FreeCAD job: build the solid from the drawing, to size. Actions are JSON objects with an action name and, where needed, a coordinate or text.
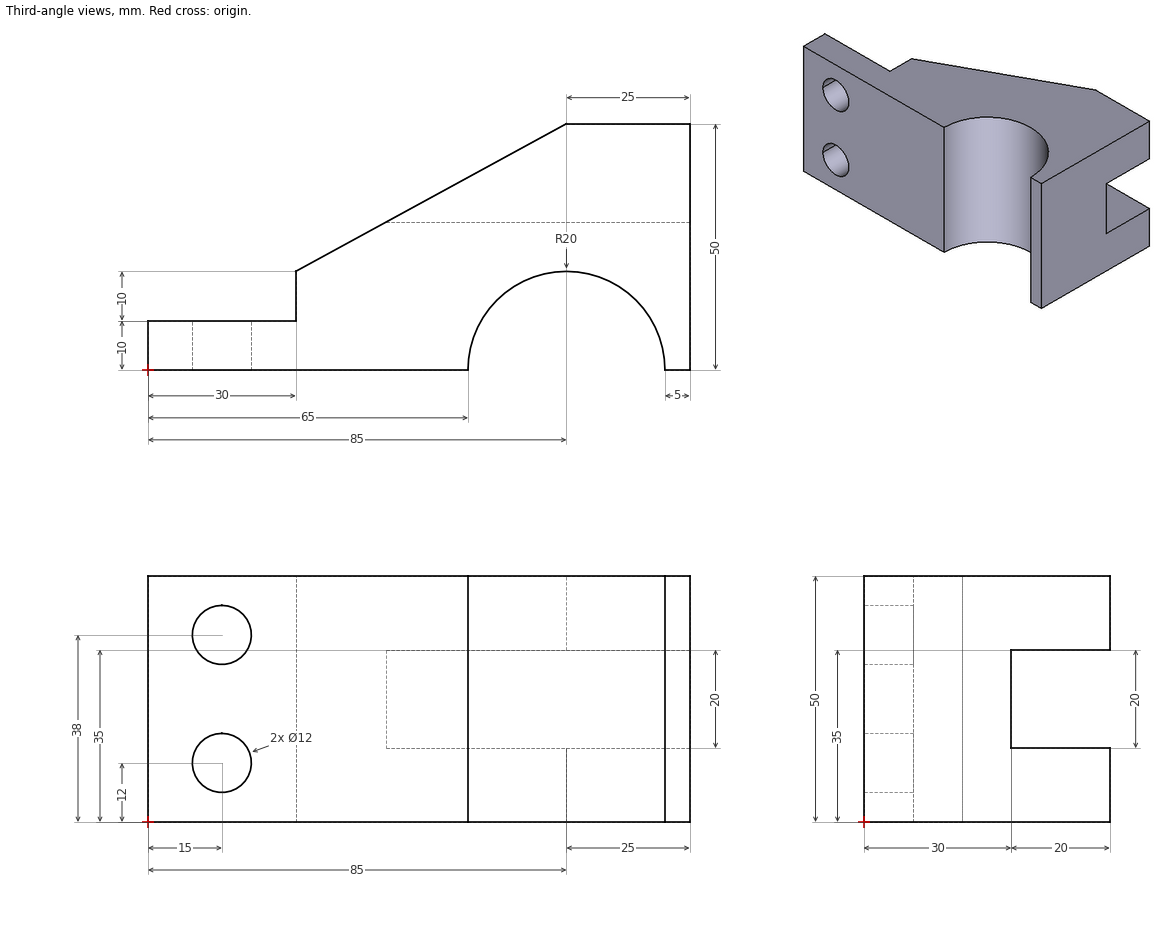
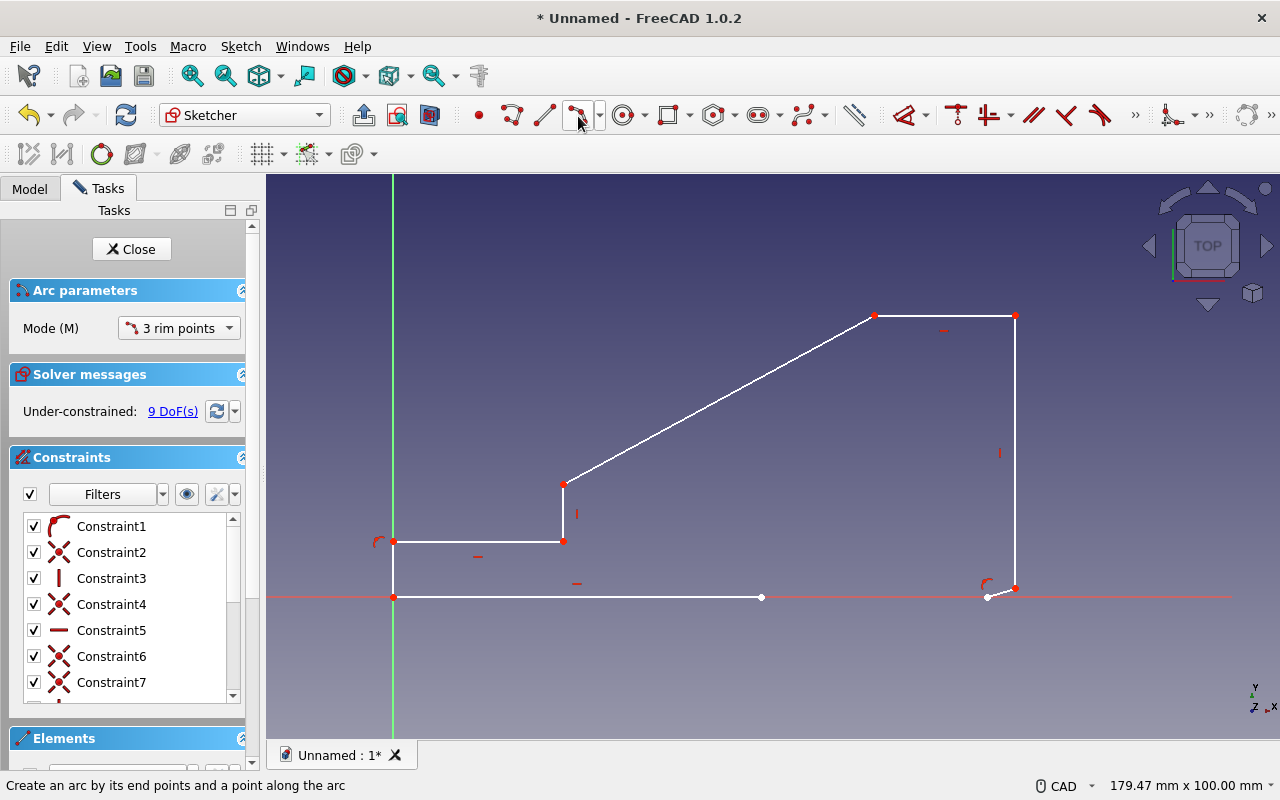
{"action": "left_click", "coordinate": [761, 588]}
{"action": "left_click", "coordinate": [987, 597]}
{"action": "left_click", "coordinate": [874, 484]}
{"action": "key", "text": "Escape"}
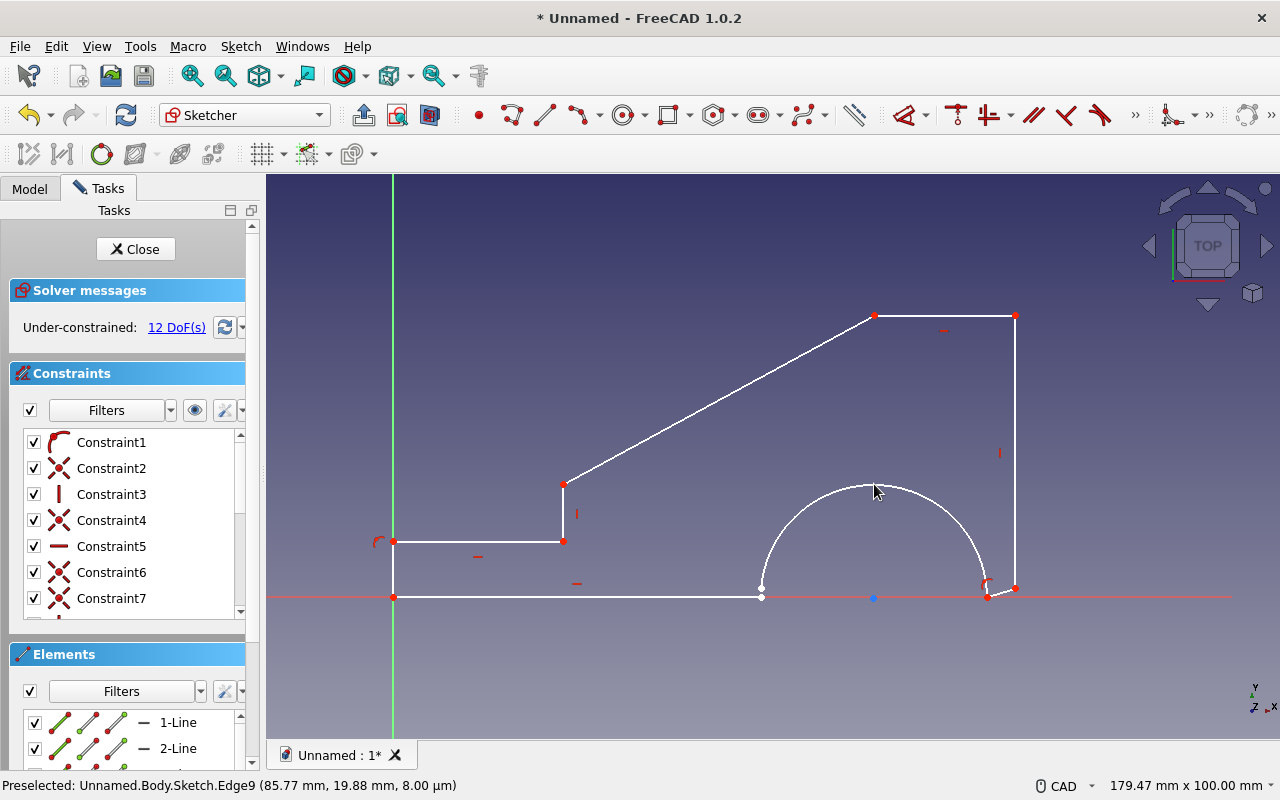
{"action": "scroll", "coordinate": [998, 594], "scroll_direction": "up", "scroll_amount": 2}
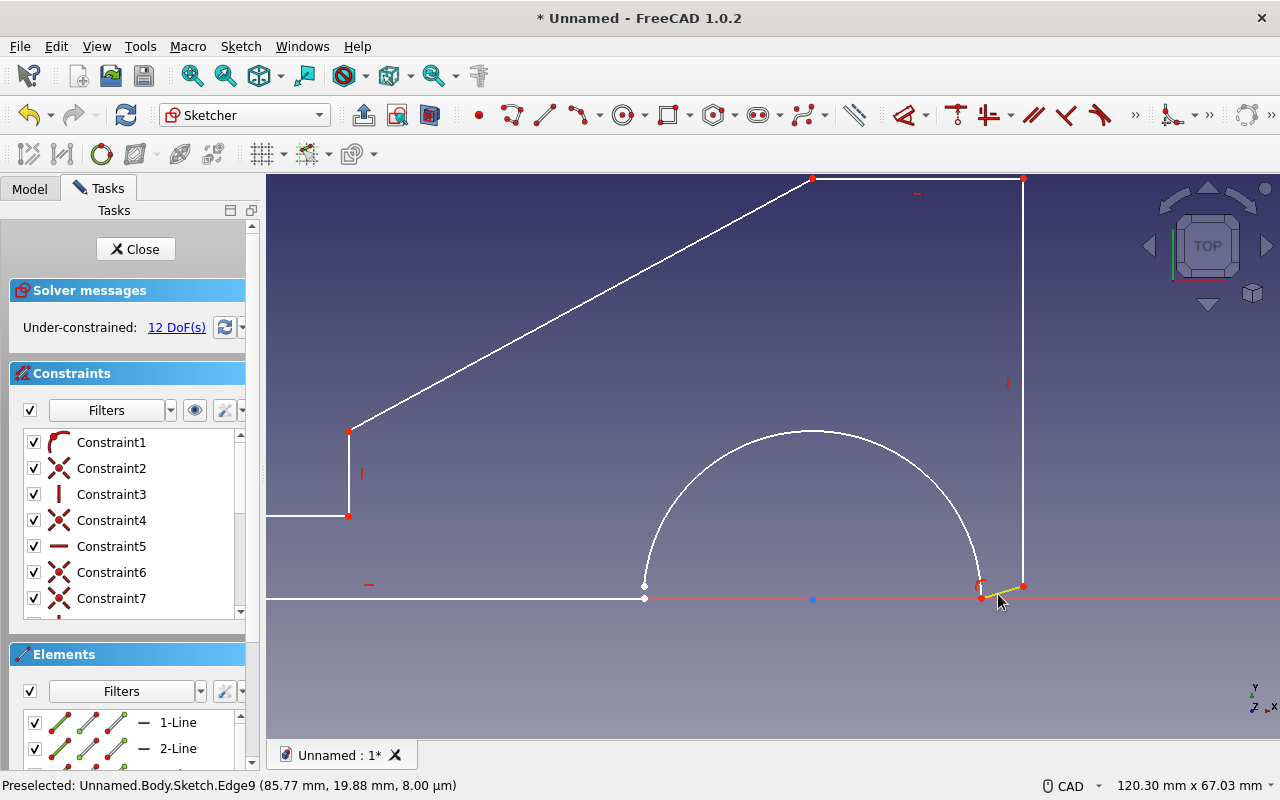
{"action": "left_click", "coordinate": [998, 594]}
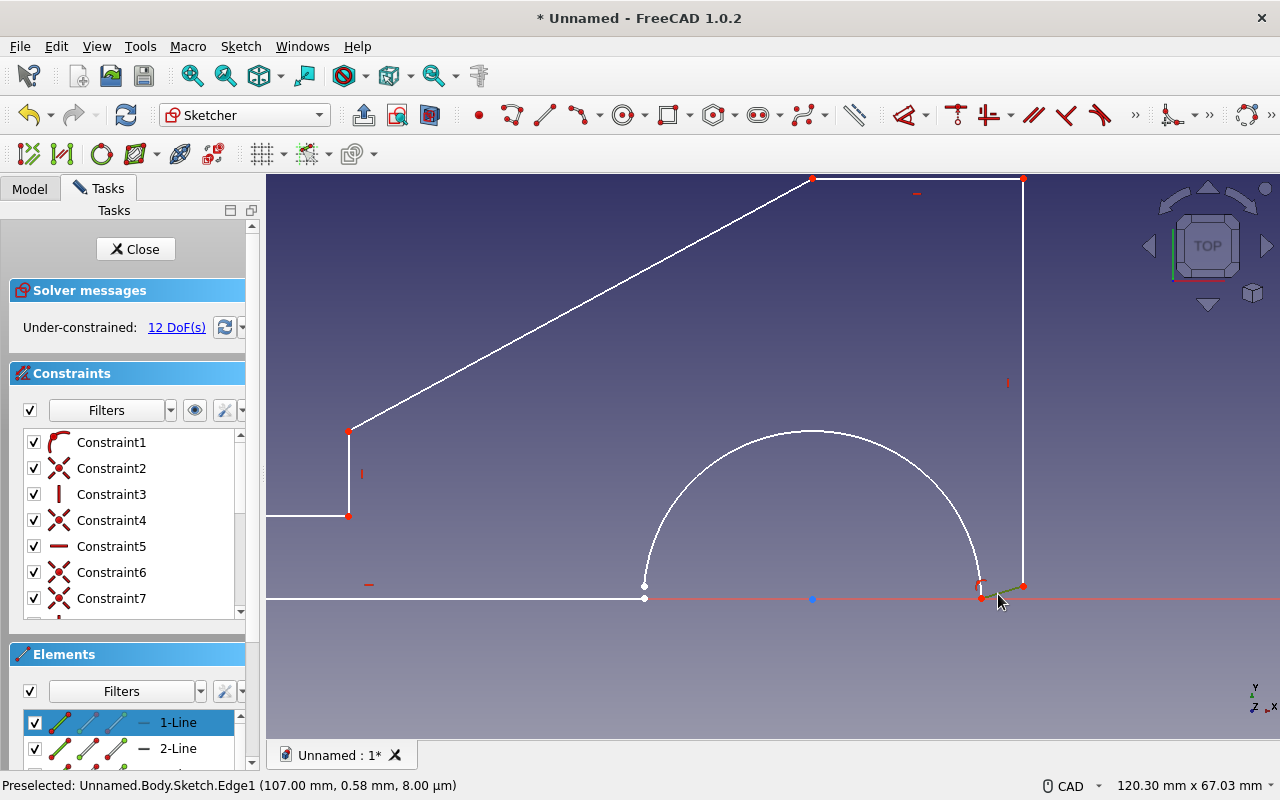
{"action": "left_click", "coordinate": [1010, 116]}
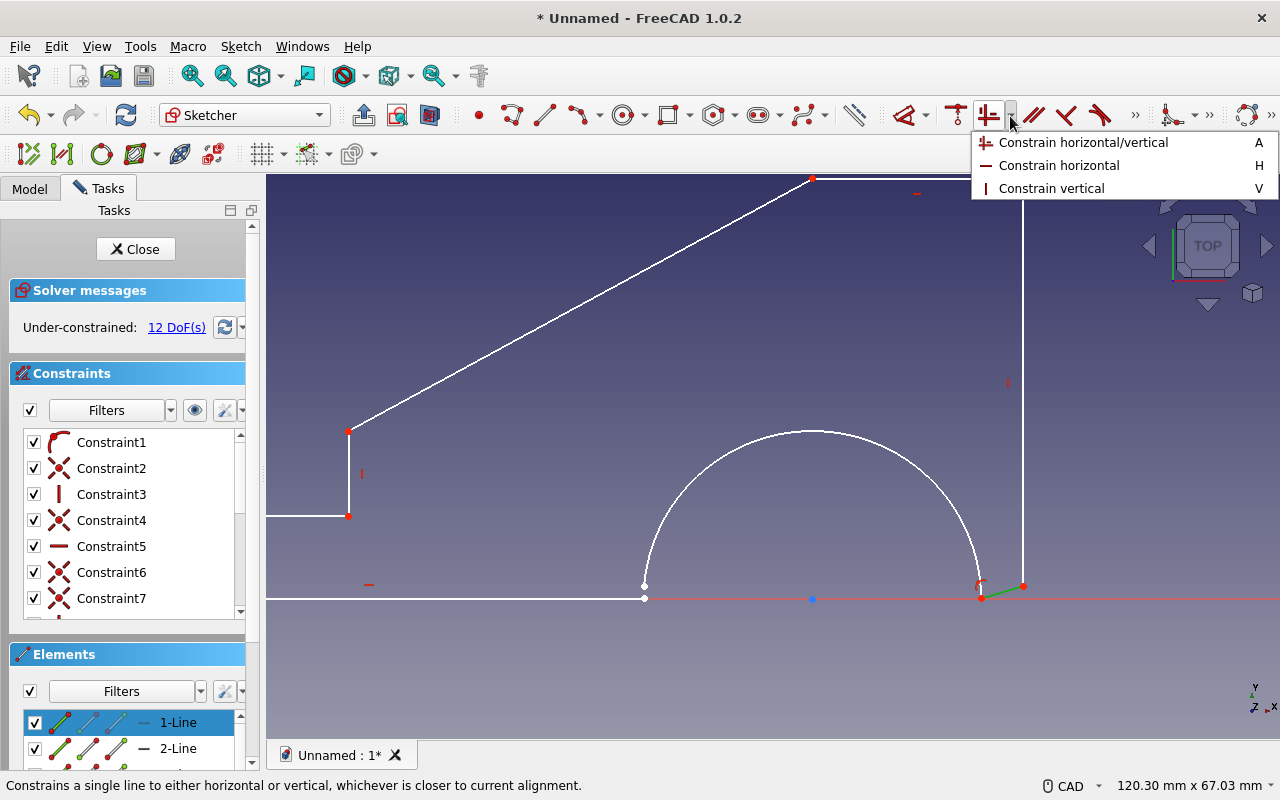
{"action": "left_click", "coordinate": [1125, 166]}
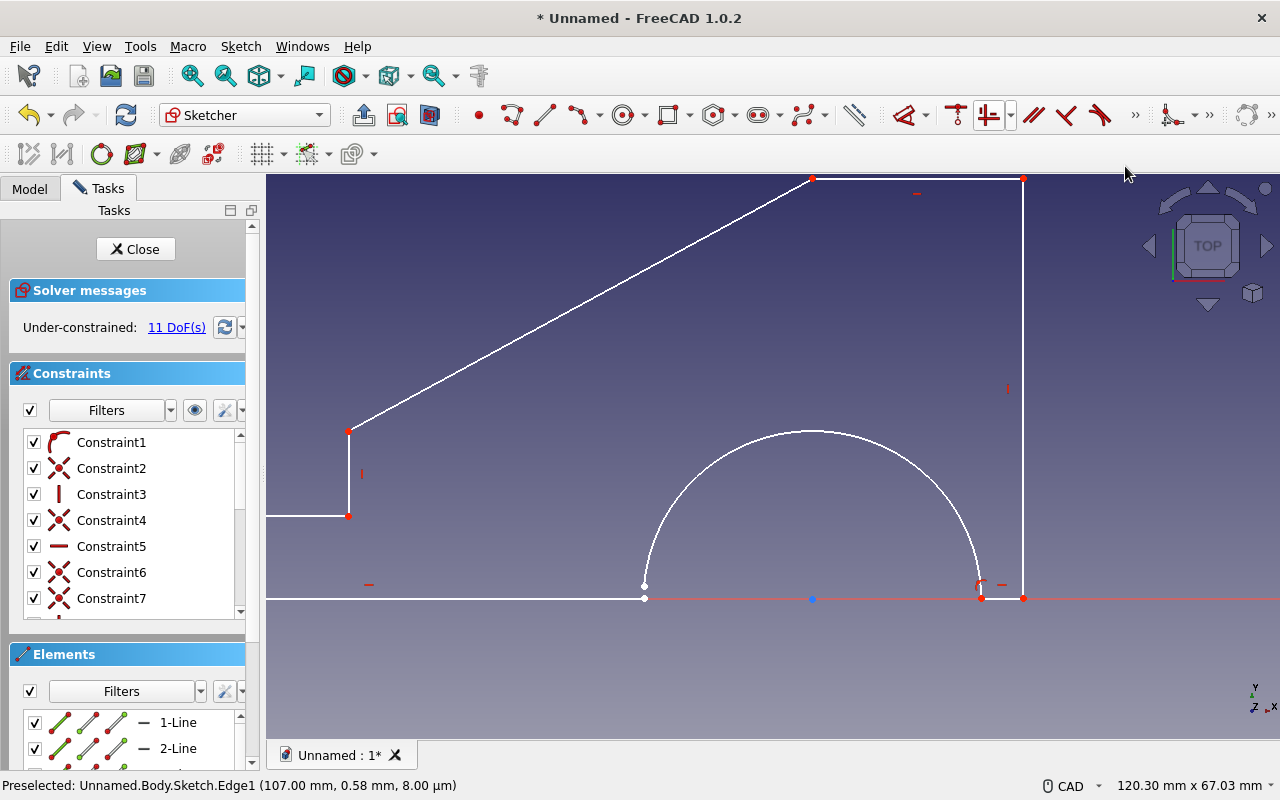
{"action": "left_click", "coordinate": [812, 600]}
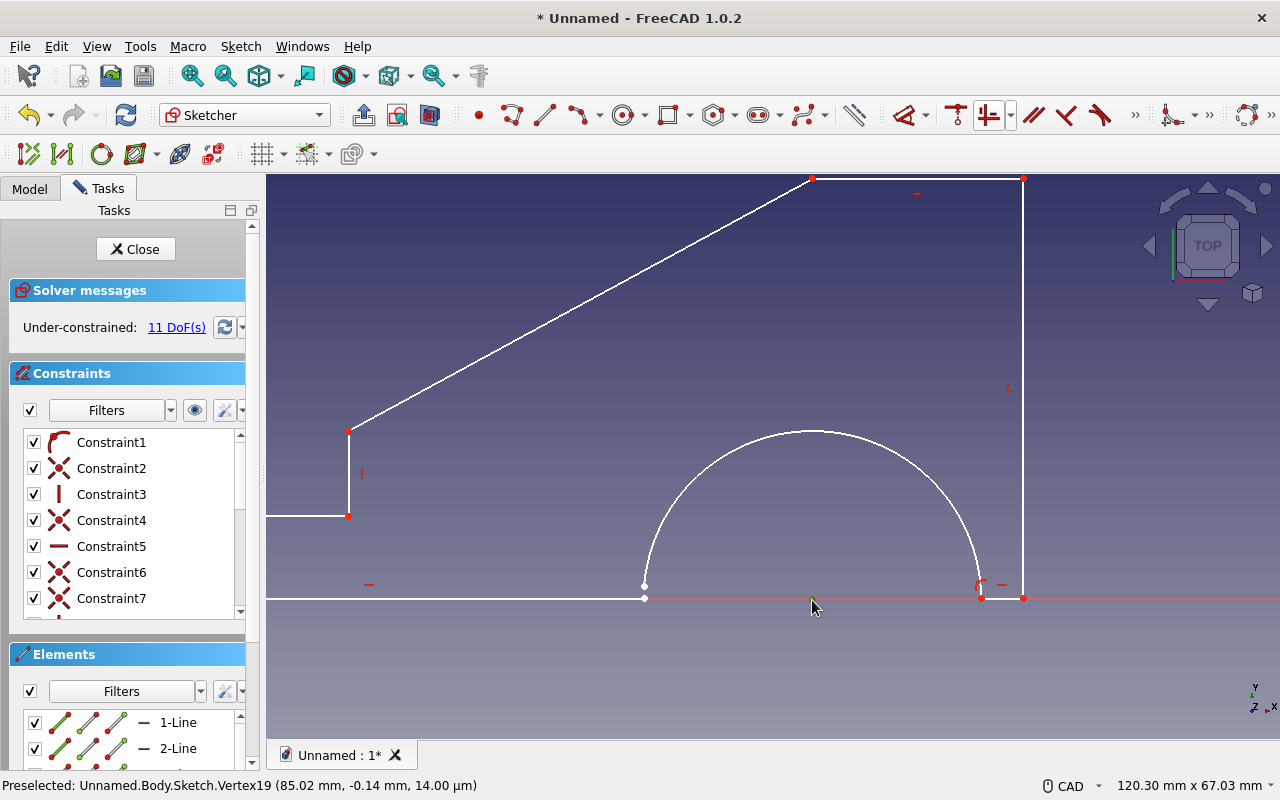
{"action": "left_click", "coordinate": [704, 599]}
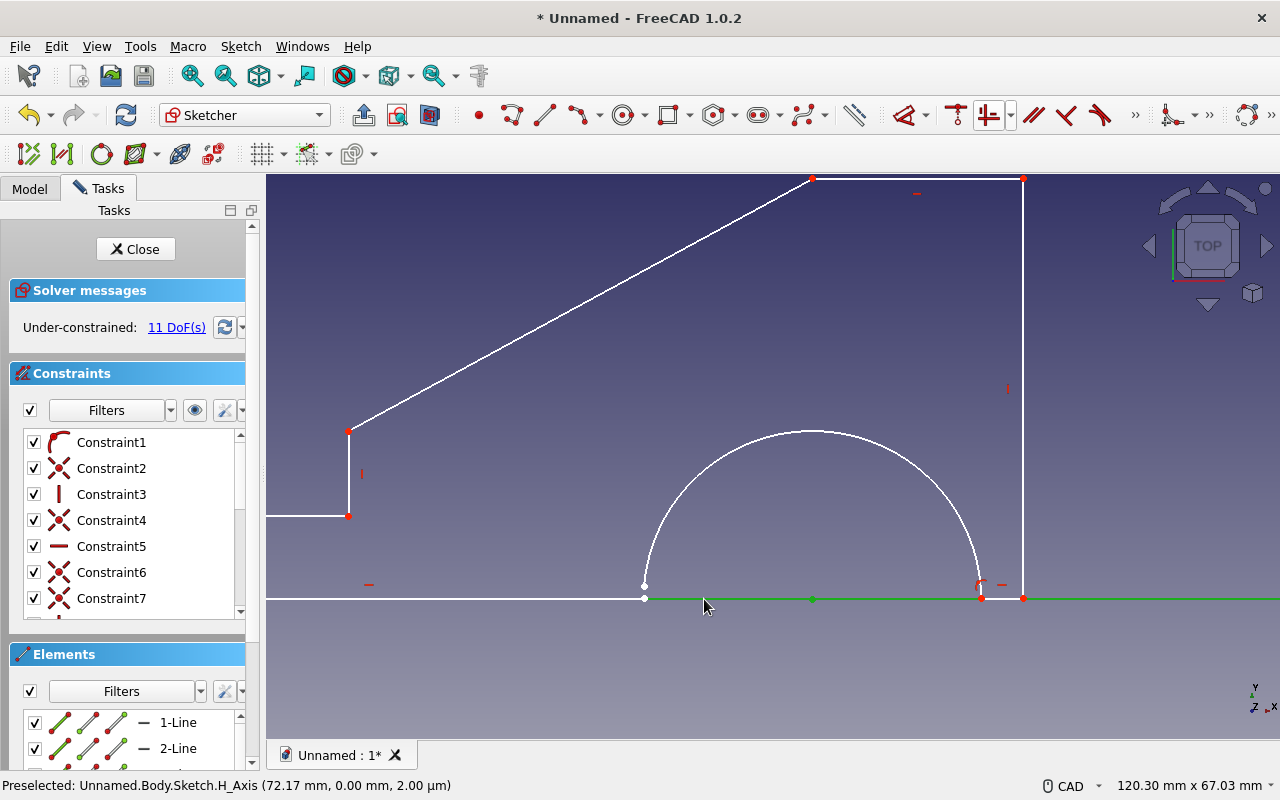
{"action": "left_click", "coordinate": [956, 116]}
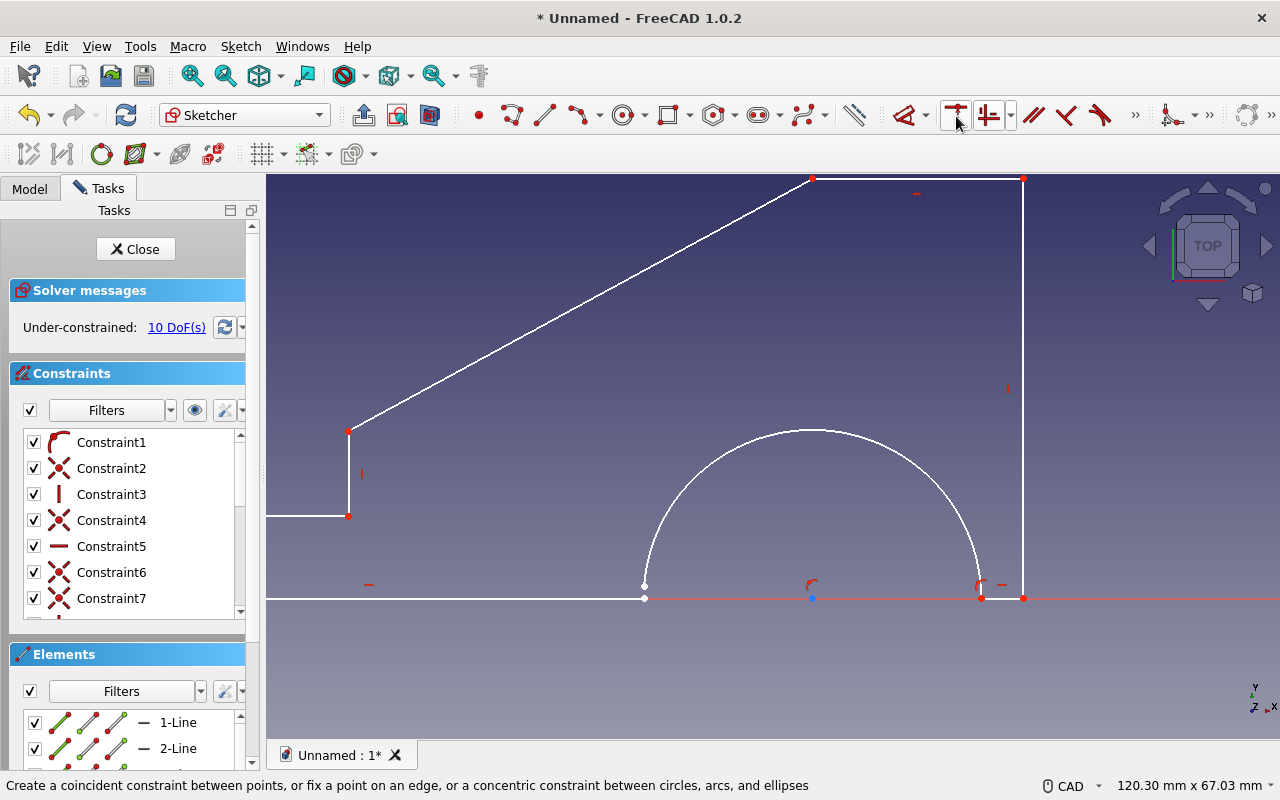
{"action": "left_click", "coordinate": [904, 116]}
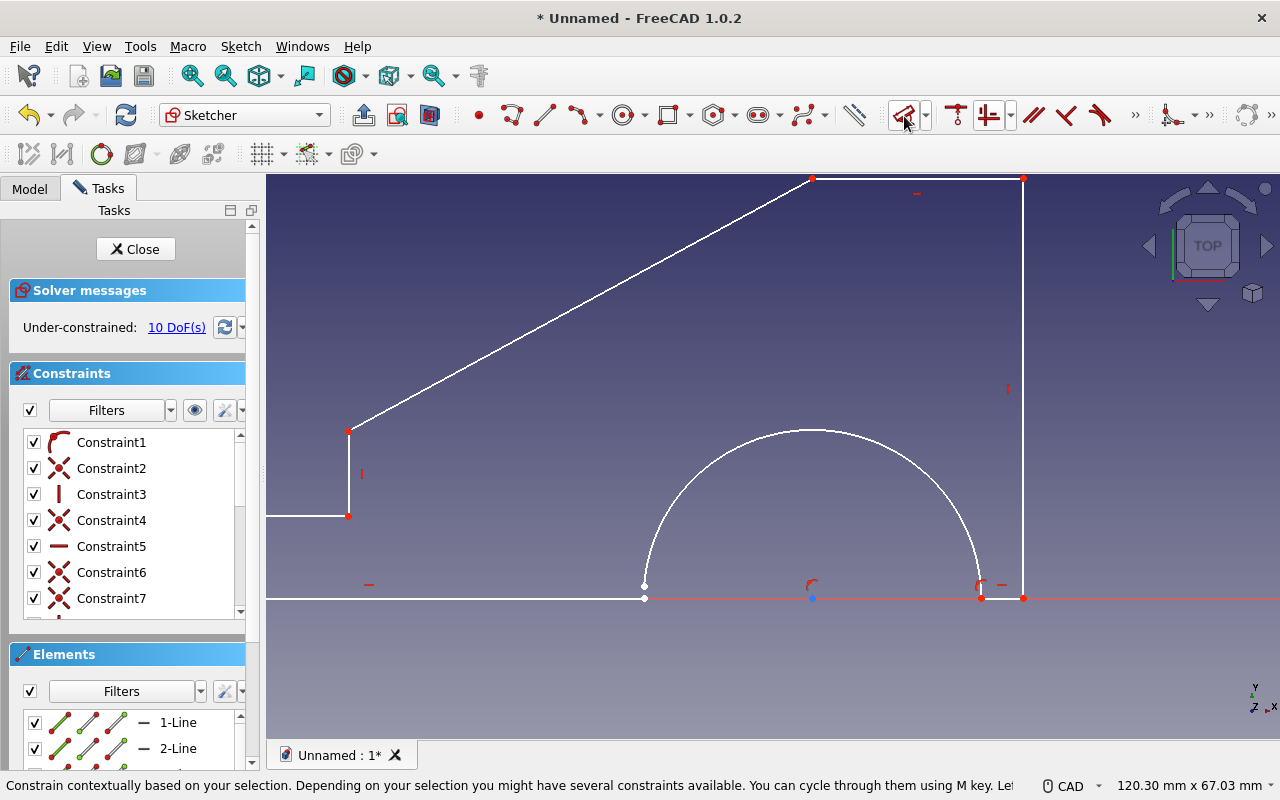
{"action": "left_click", "coordinate": [915, 464]}
{"action": "left_click", "coordinate": [934, 439]}